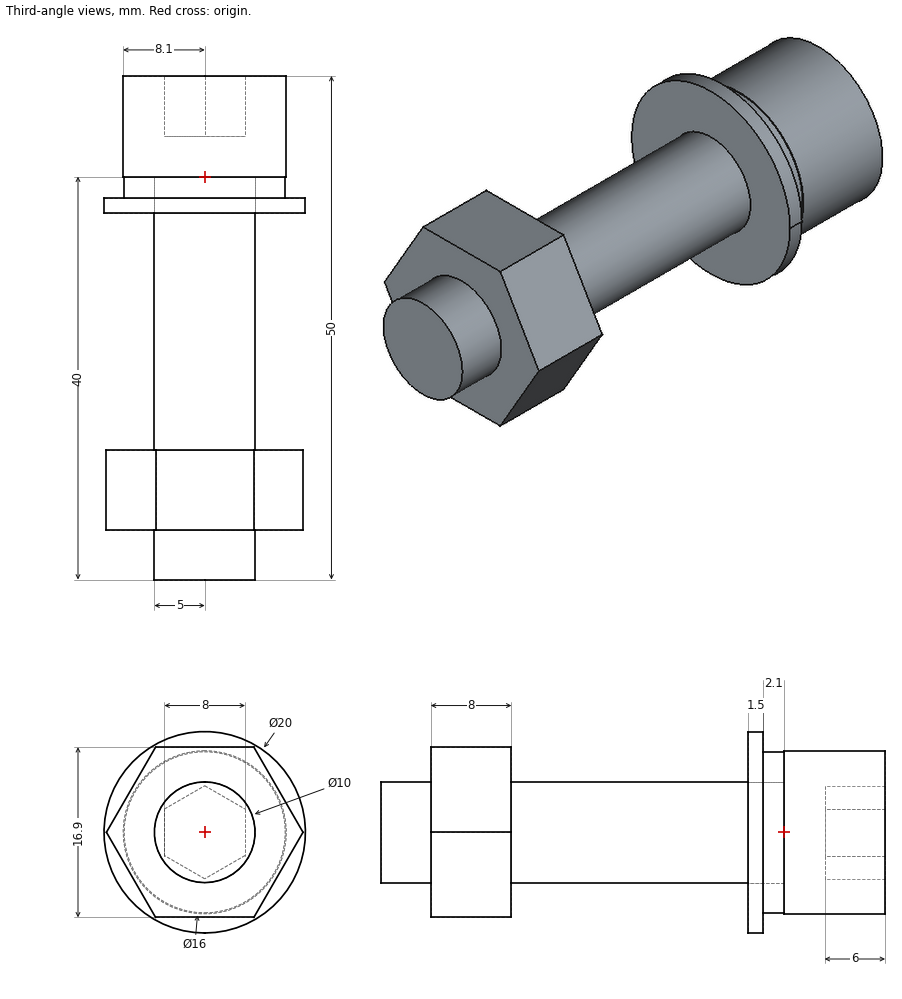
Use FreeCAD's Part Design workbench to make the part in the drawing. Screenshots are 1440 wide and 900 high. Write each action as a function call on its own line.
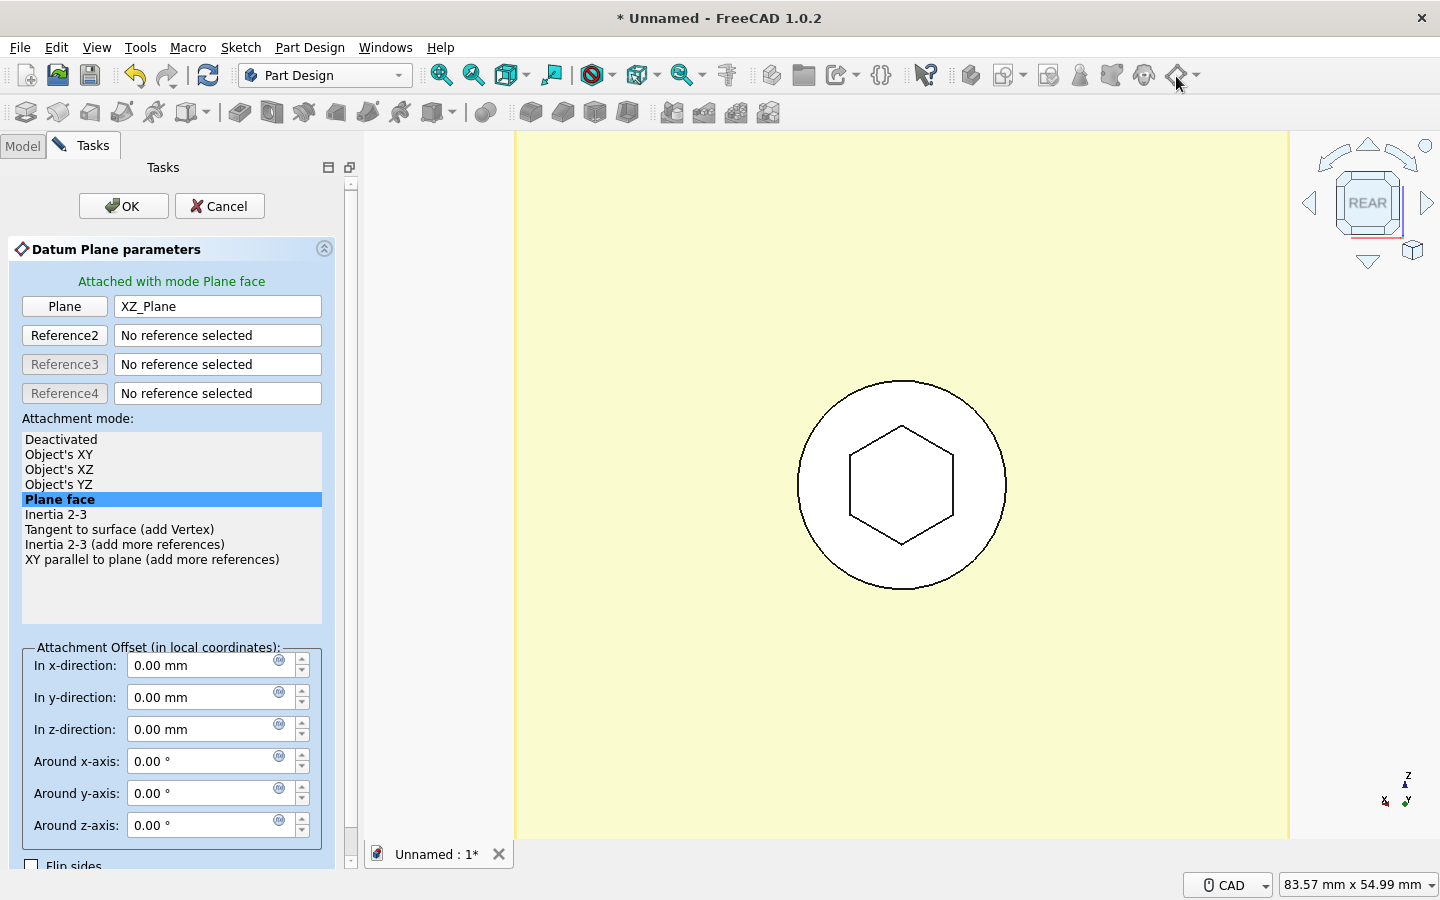
triple_click(210, 729)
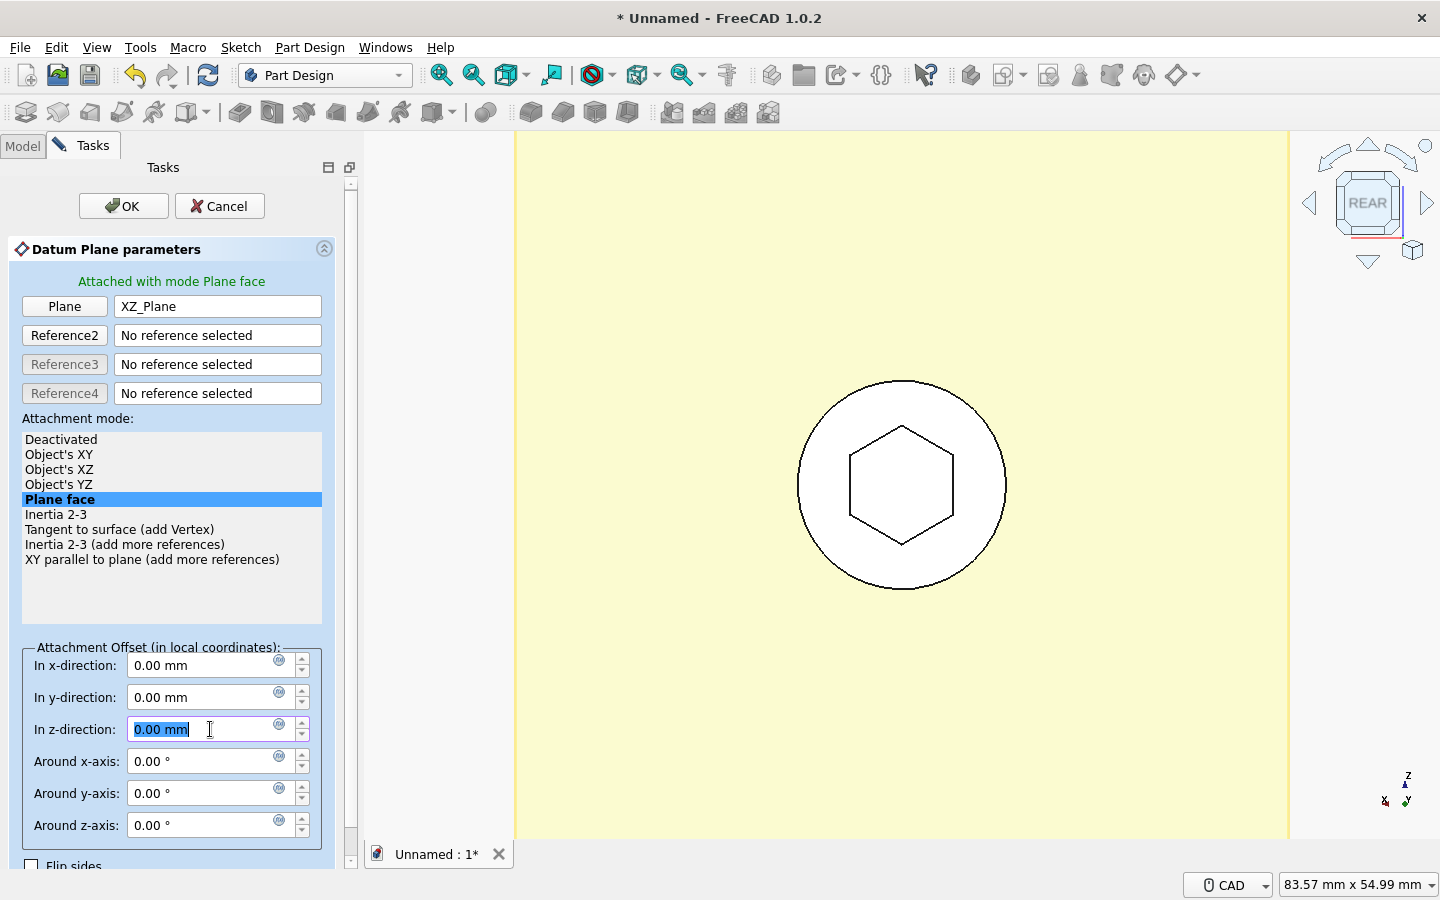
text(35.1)
key(Tab)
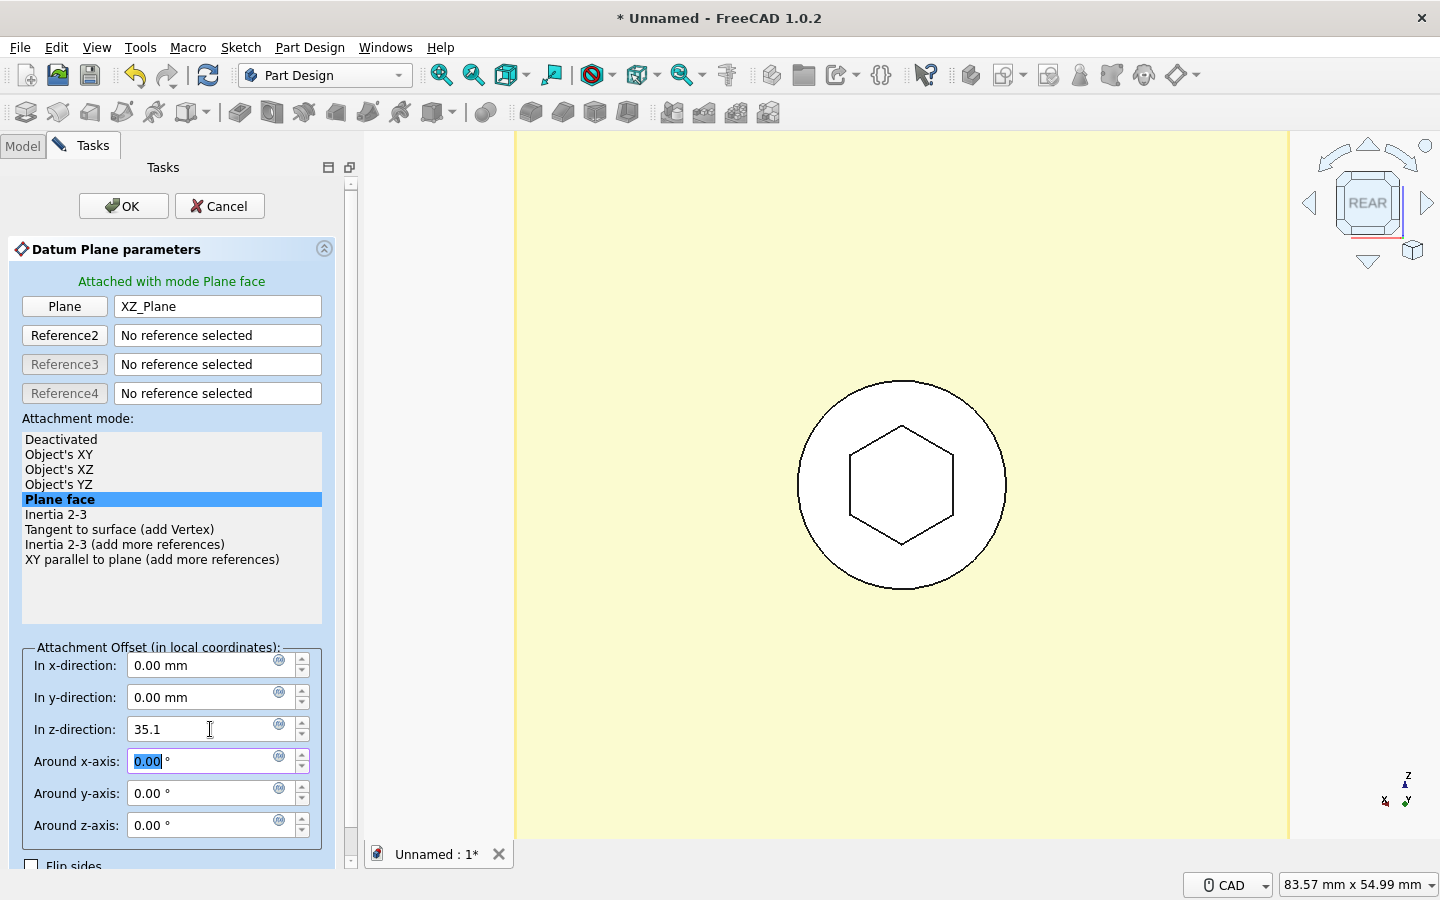
click(124, 206)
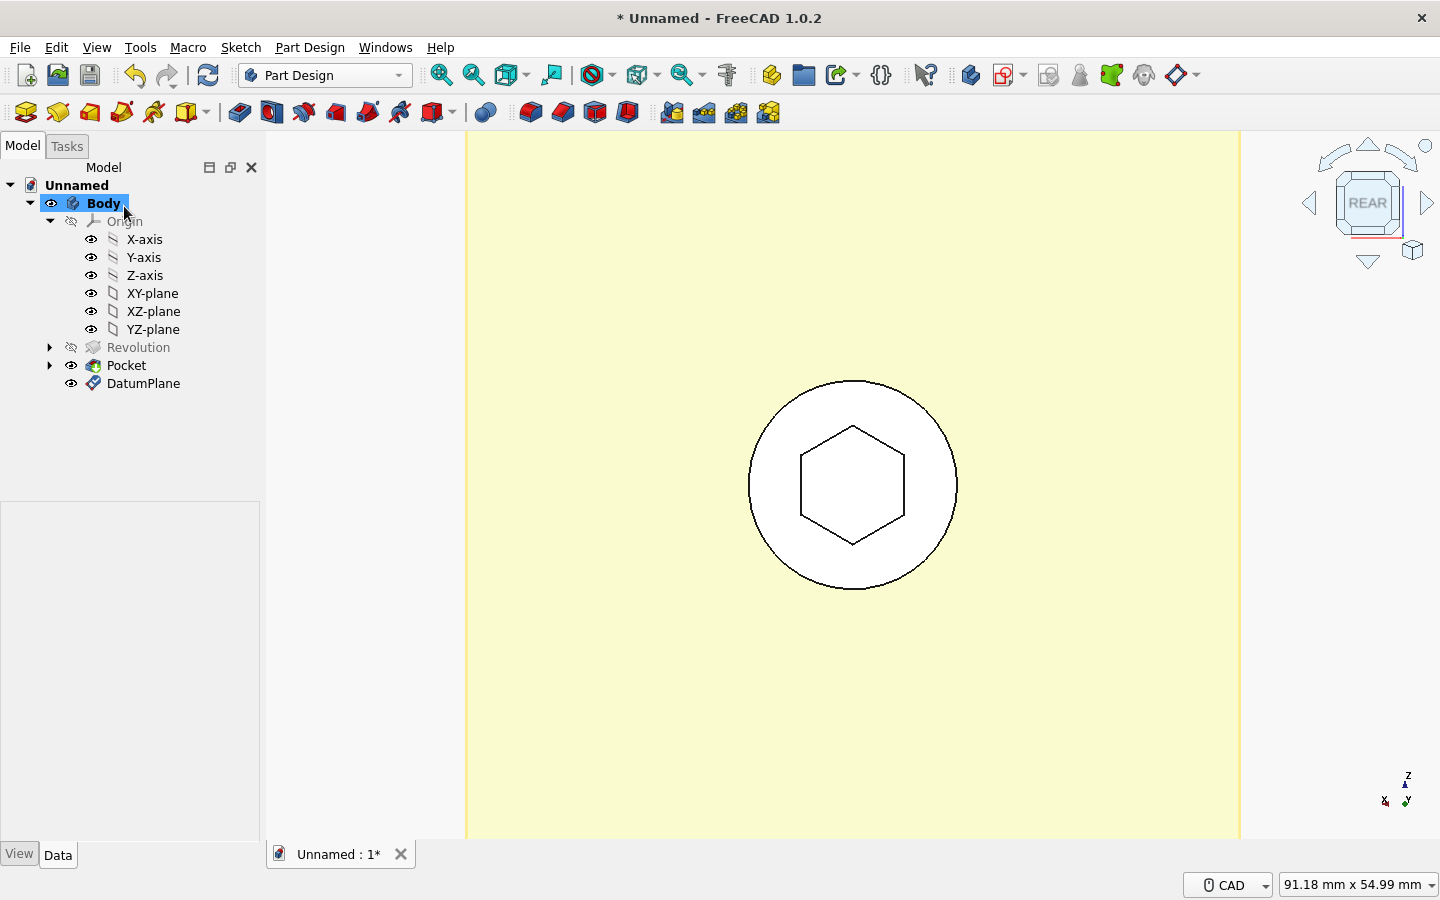
click(116, 383)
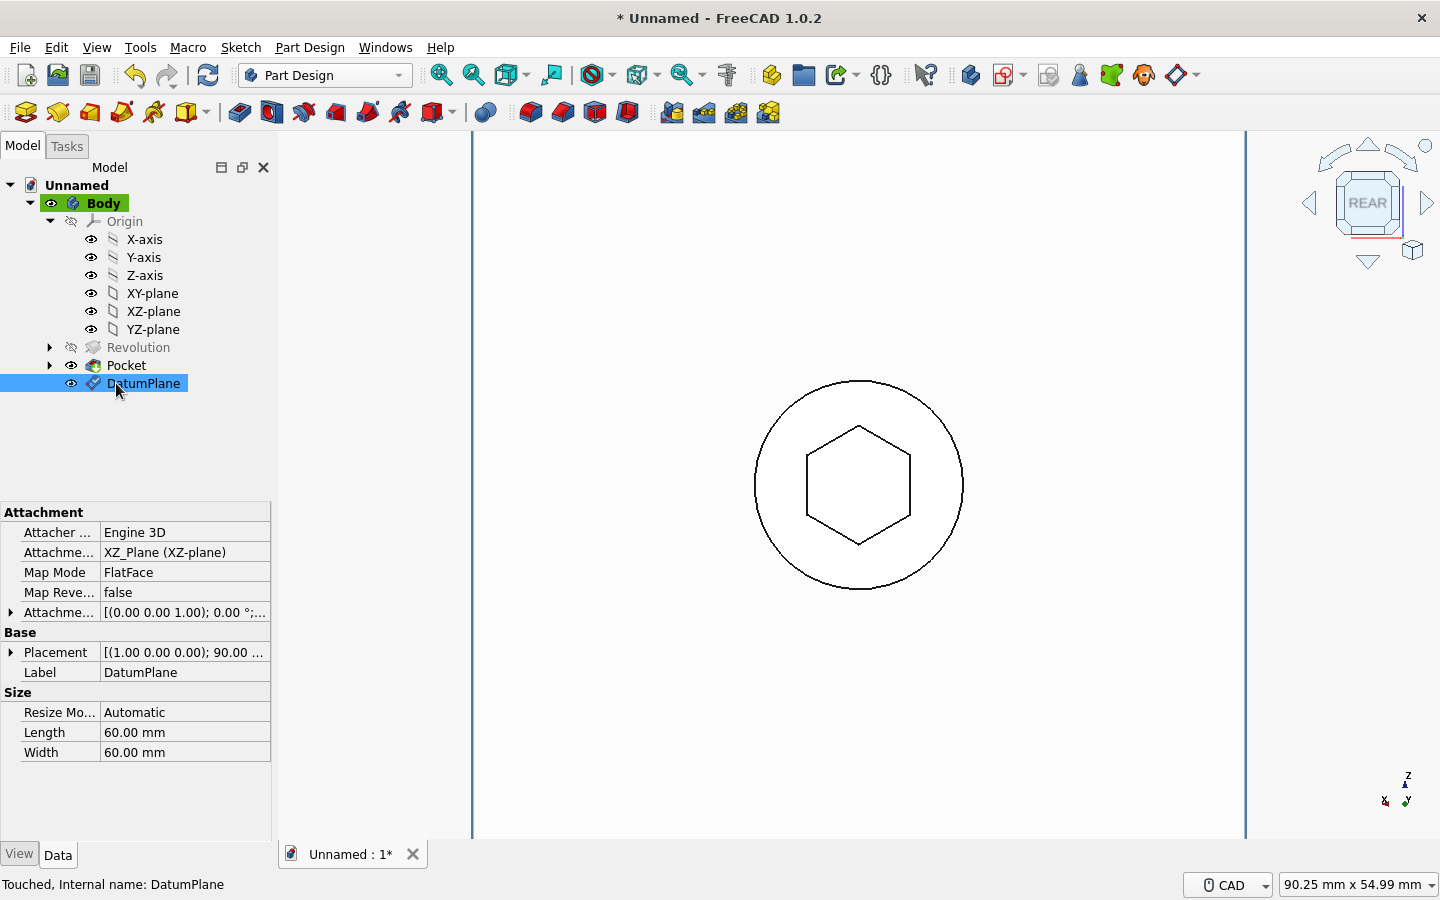
click(1004, 76)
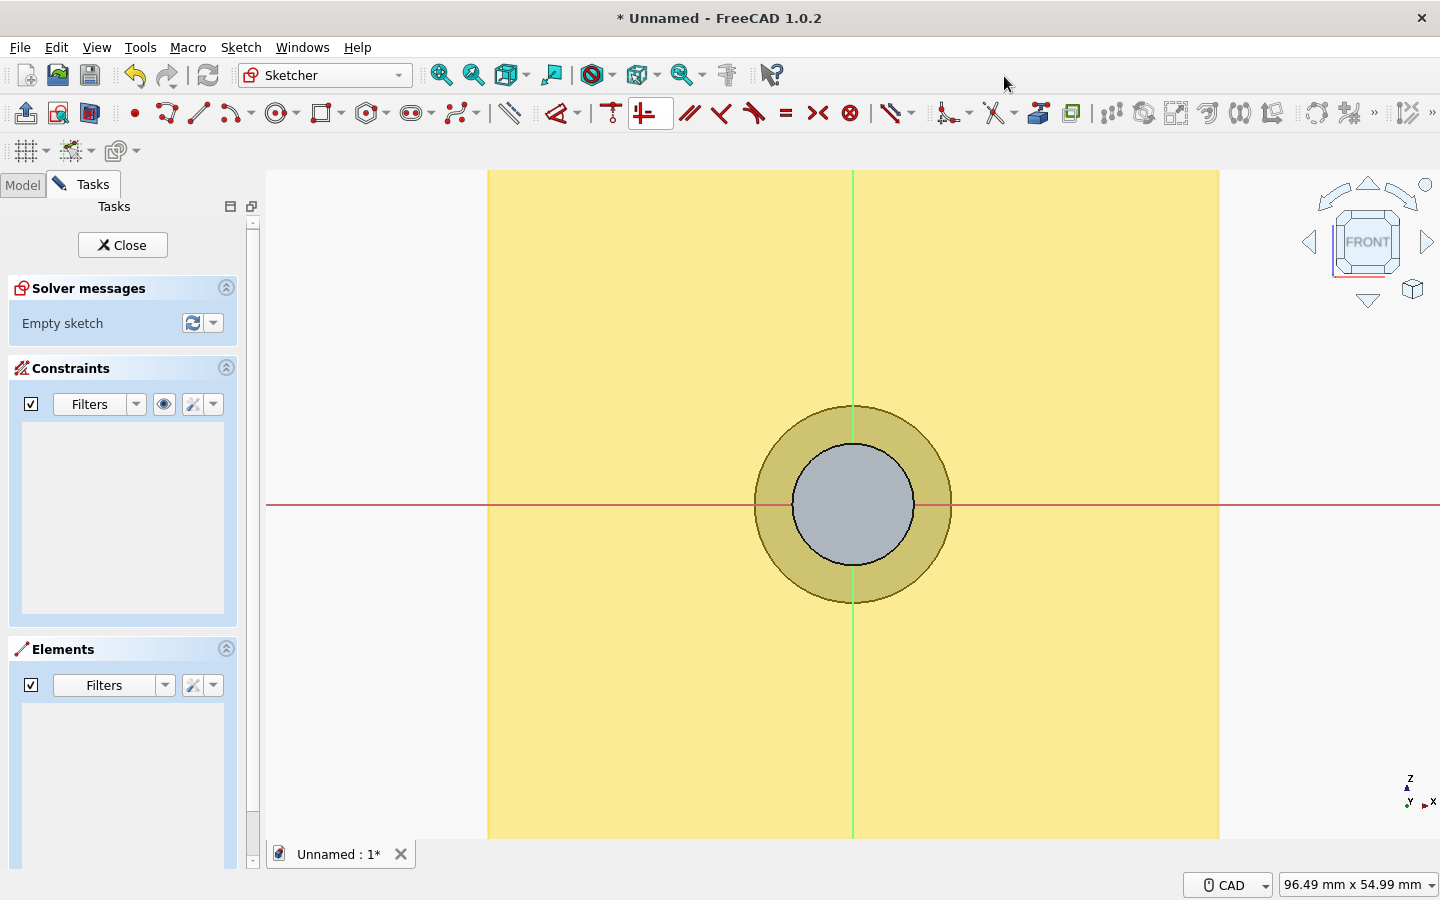
click(90, 114)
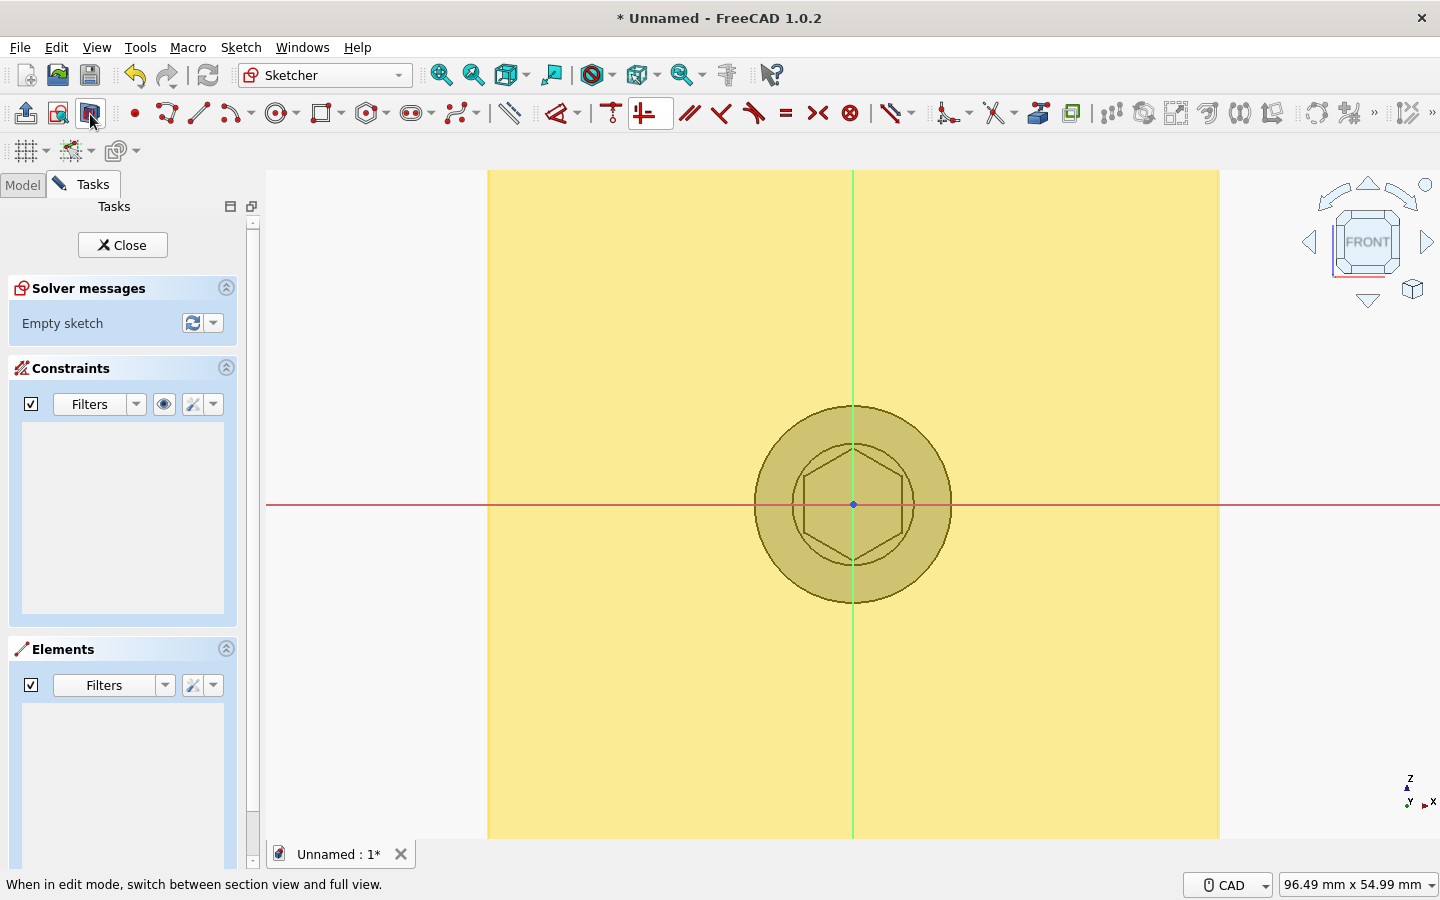
scroll(909, 505, up, 4)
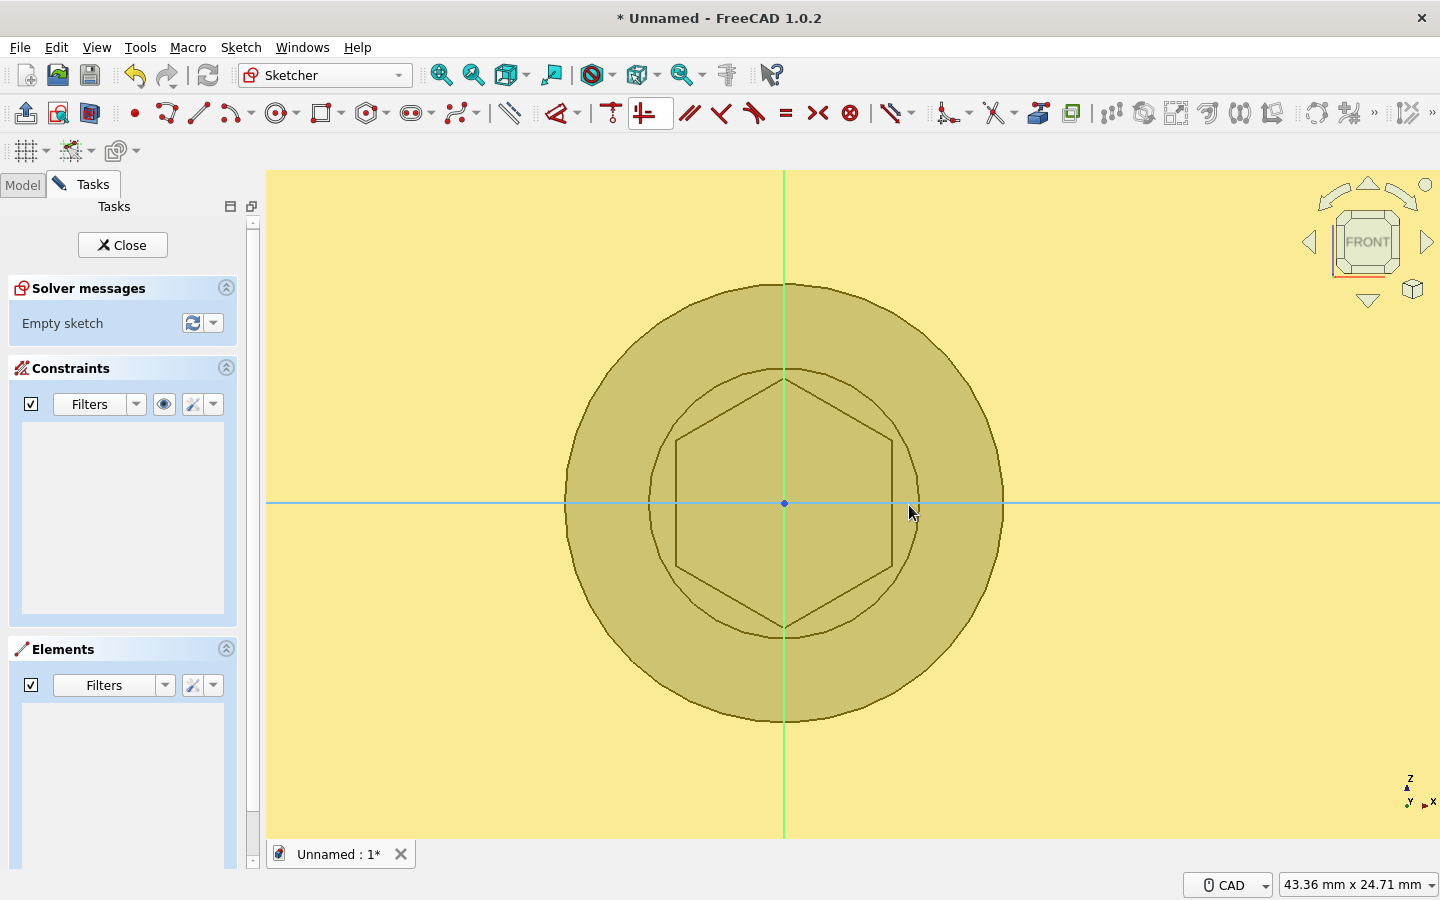
click(366, 114)